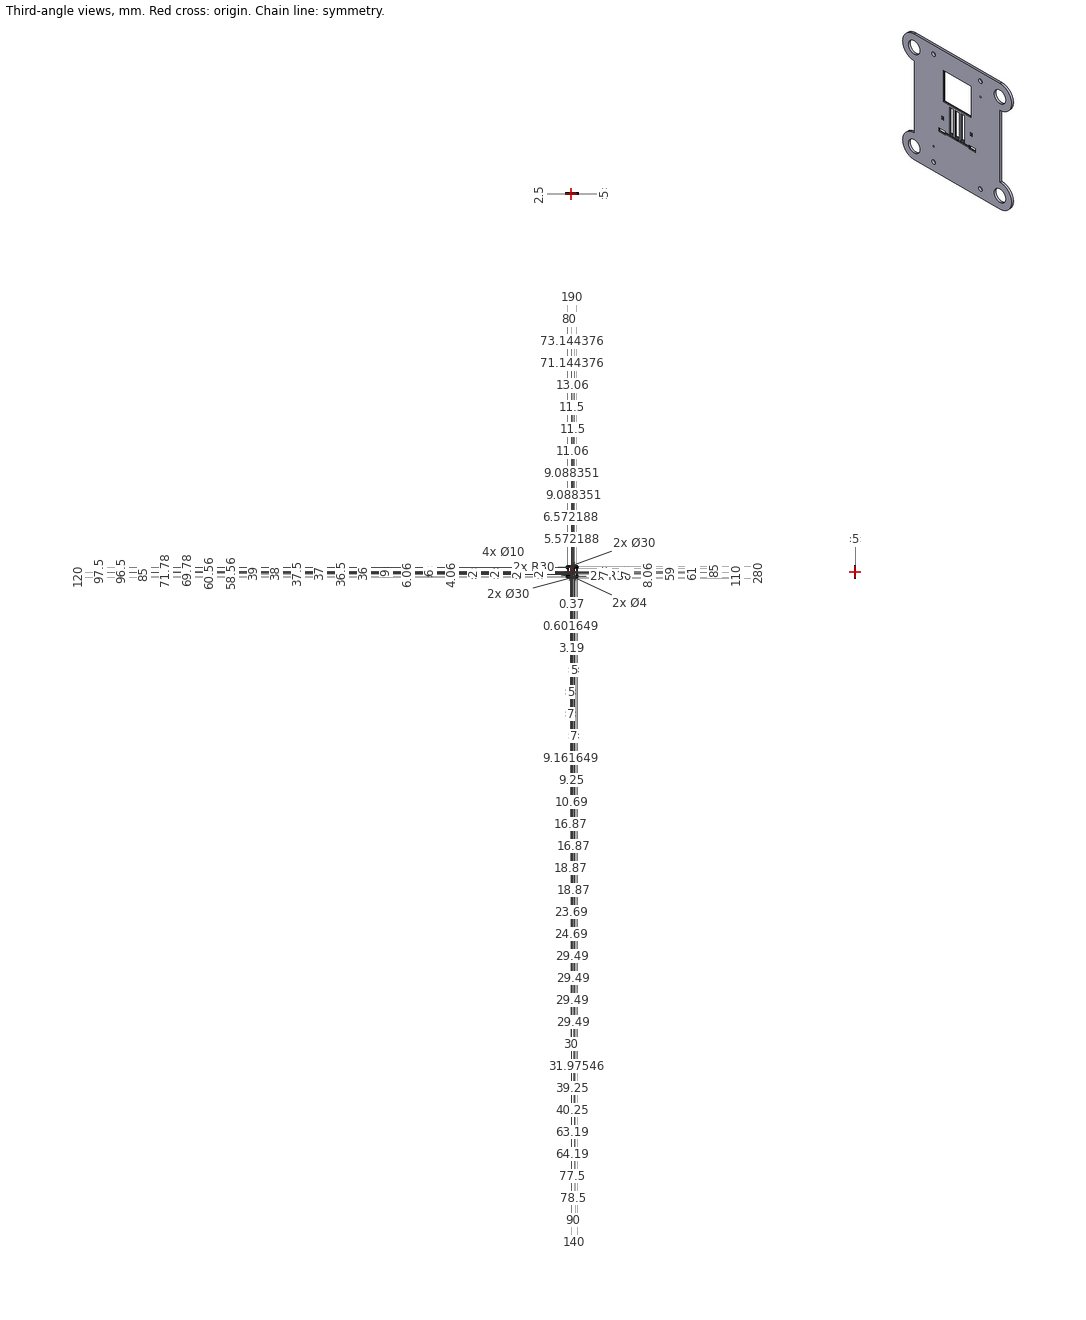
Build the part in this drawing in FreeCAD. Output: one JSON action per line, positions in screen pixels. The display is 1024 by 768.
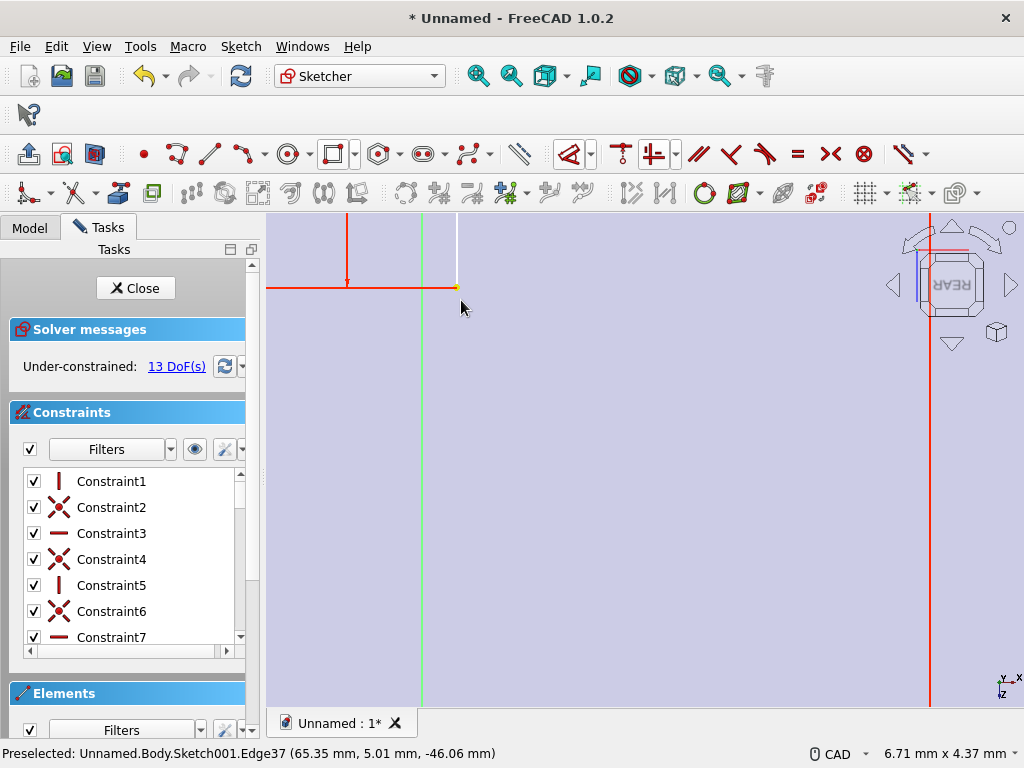
{"action": "left_click", "coordinate": [457, 288]}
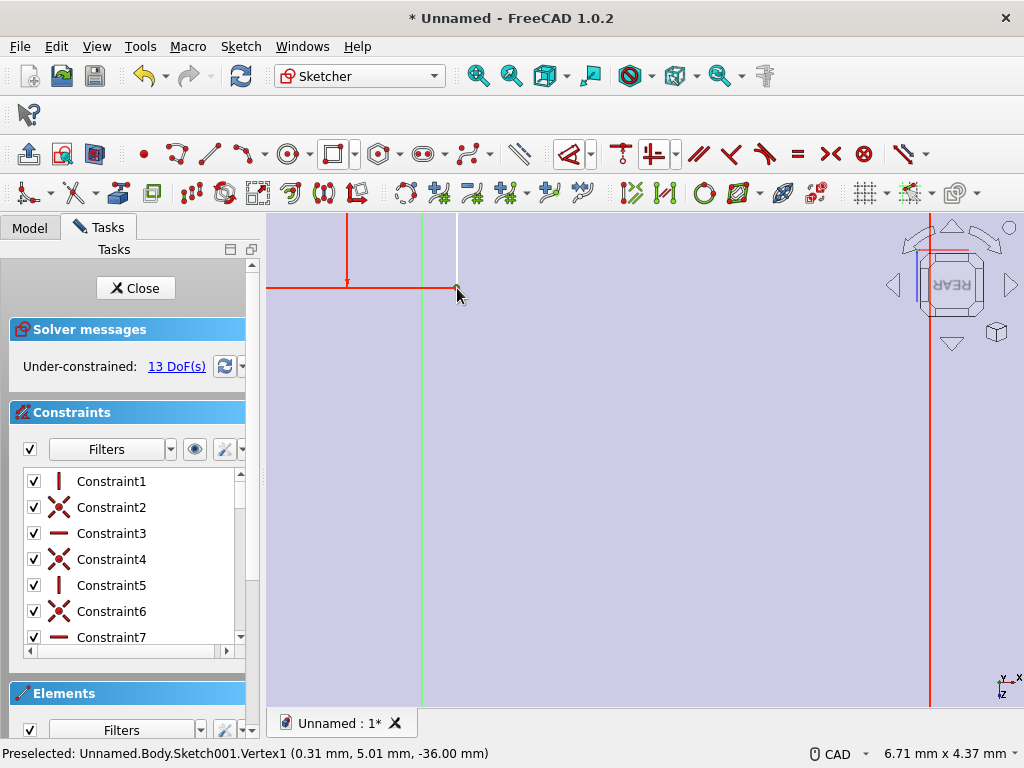
{"action": "left_click", "coordinate": [590, 154]}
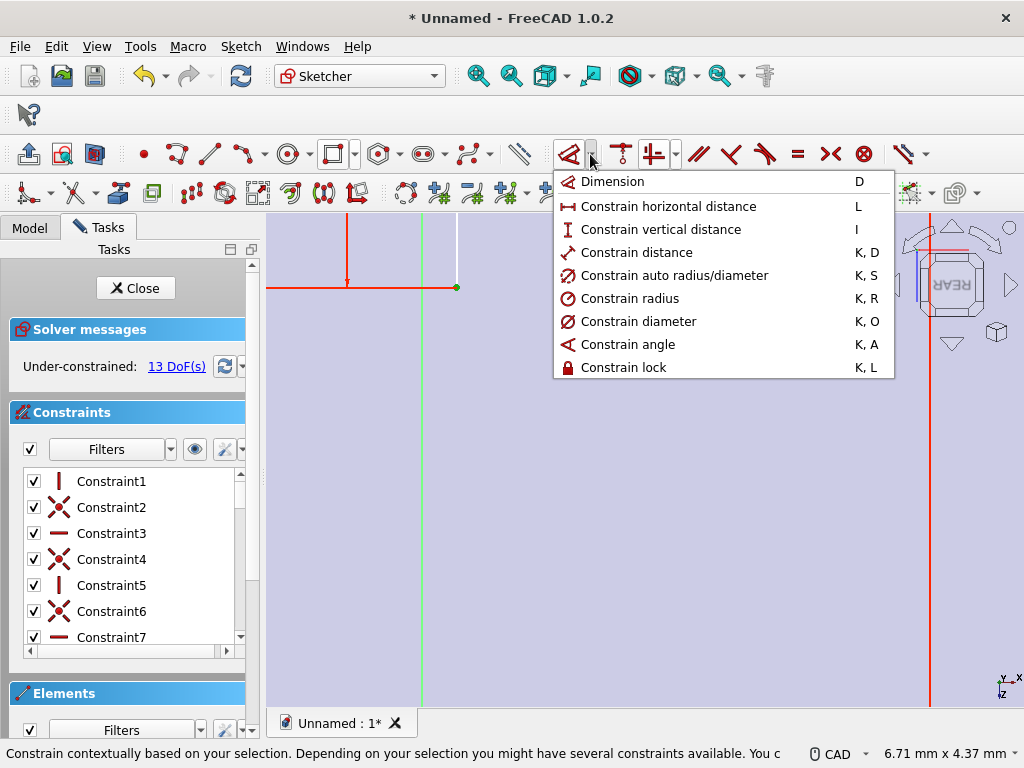
{"action": "left_click", "coordinate": [724, 206]}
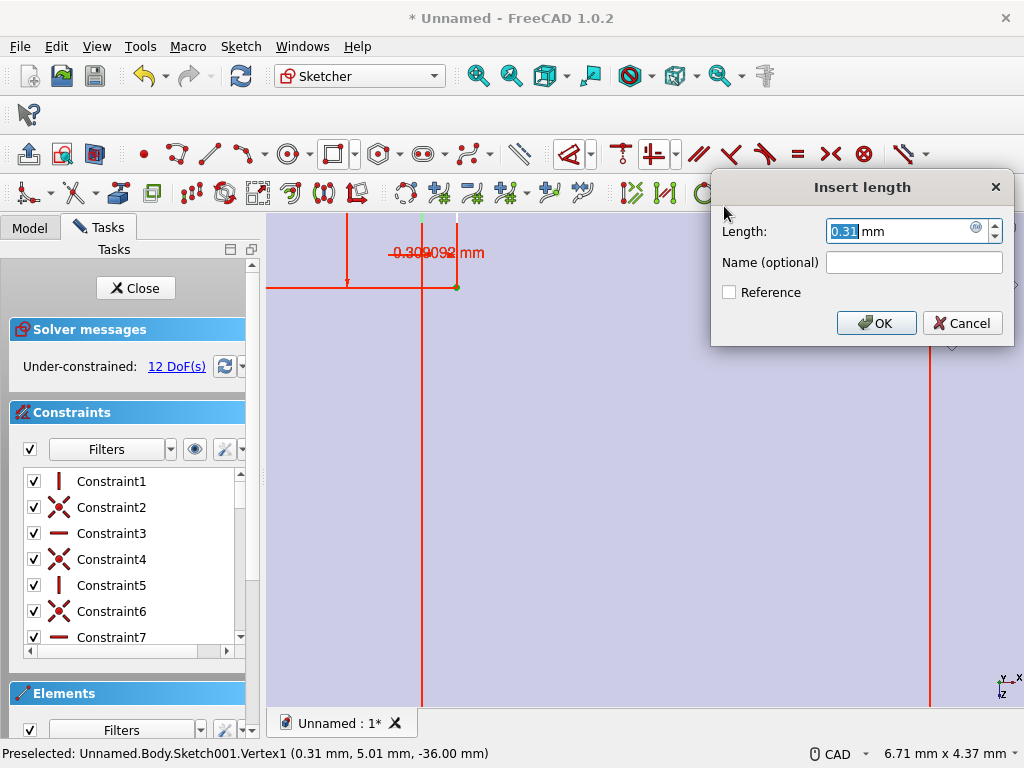
{"action": "type", "text": "0.37"}
{"action": "key", "text": "Return"}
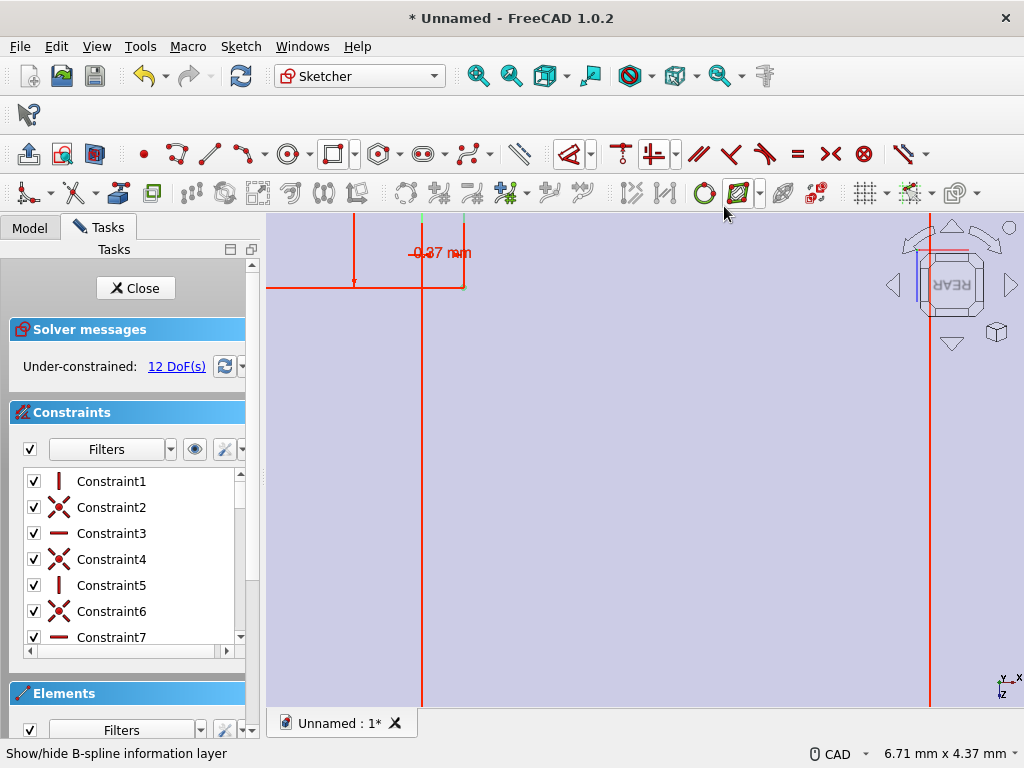
{"action": "scroll", "coordinate": [576, 460], "scroll_direction": "down", "scroll_amount": 15}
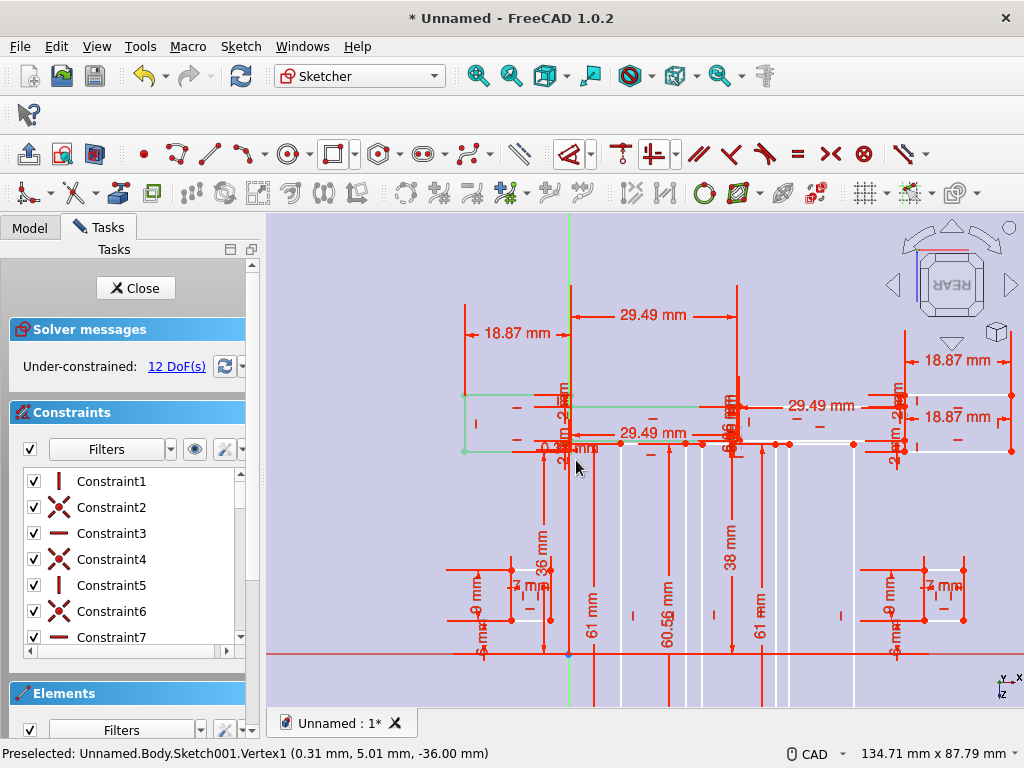
{"action": "scroll", "coordinate": [483, 263], "scroll_direction": "down", "scroll_amount": 5}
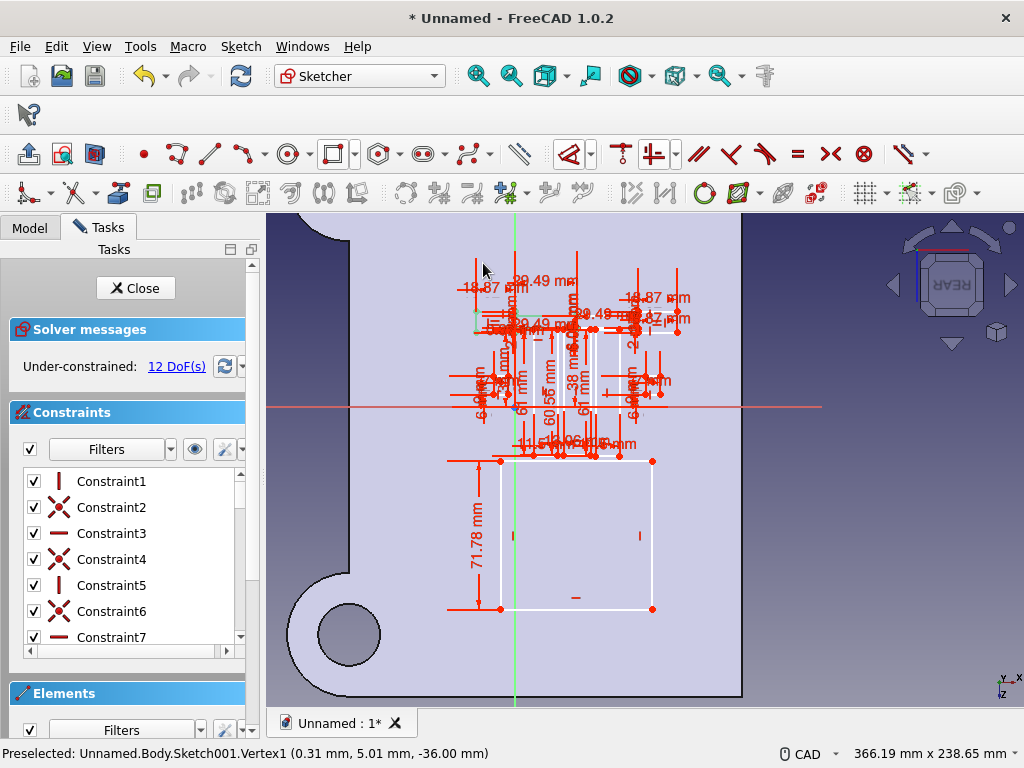
{"action": "left_click", "coordinate": [501, 610]}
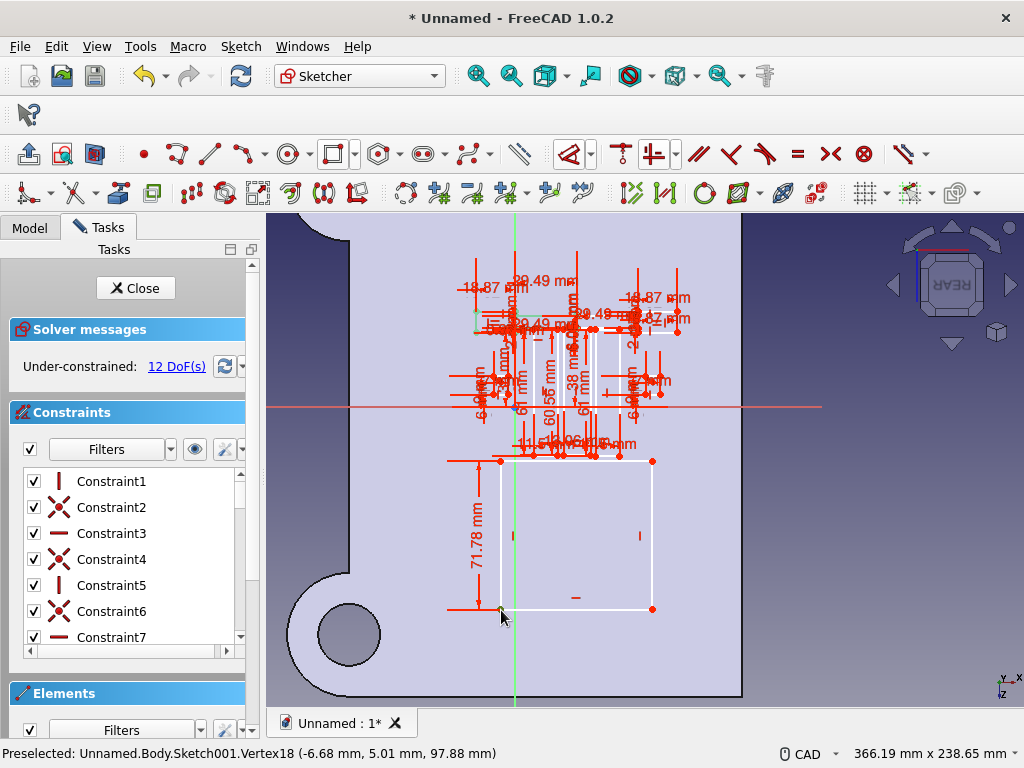
{"action": "left_click", "coordinate": [590, 154]}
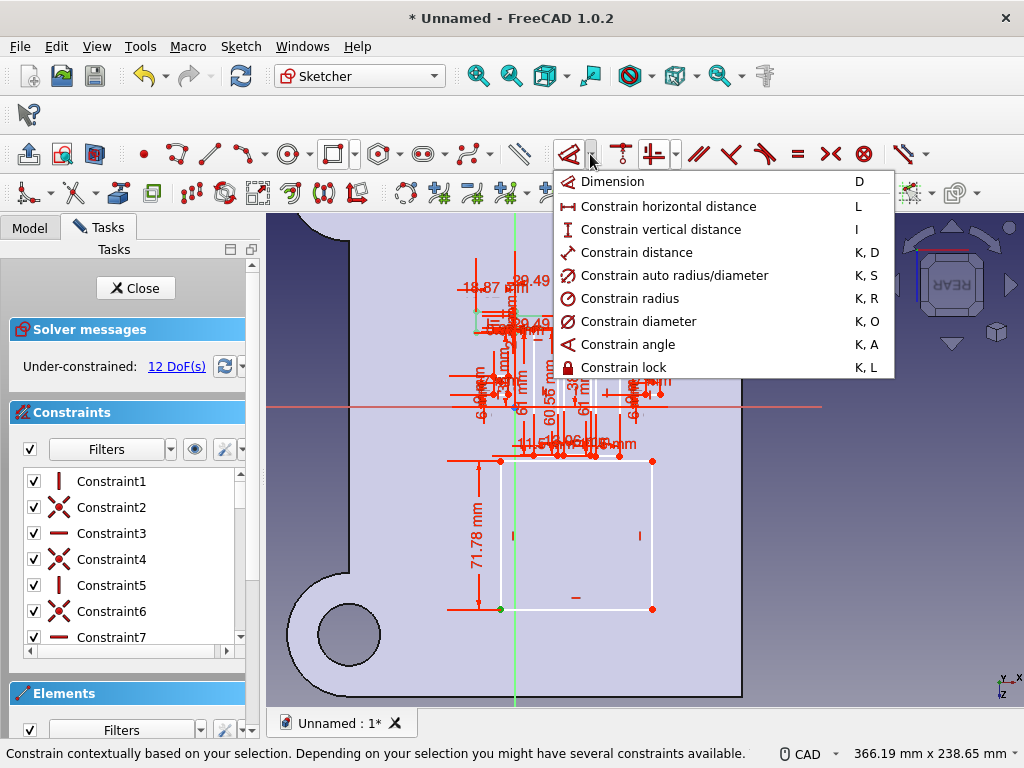
{"action": "left_click", "coordinate": [724, 230]}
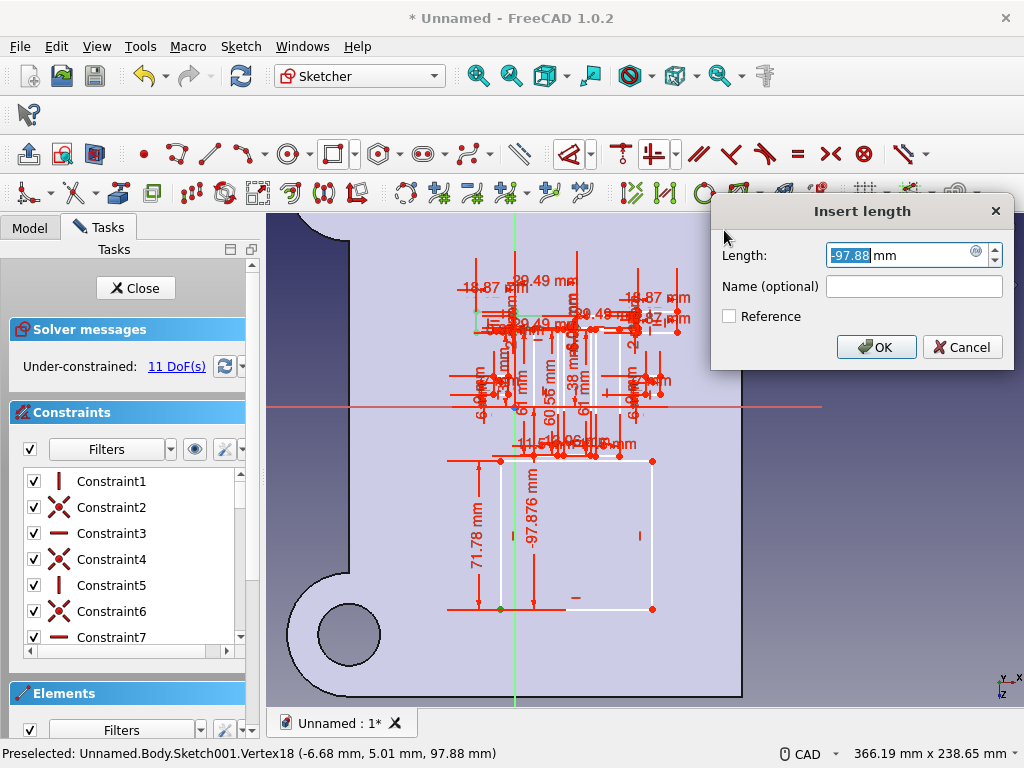
{"action": "type", "text": "-97.5"}
{"action": "key", "text": "Return"}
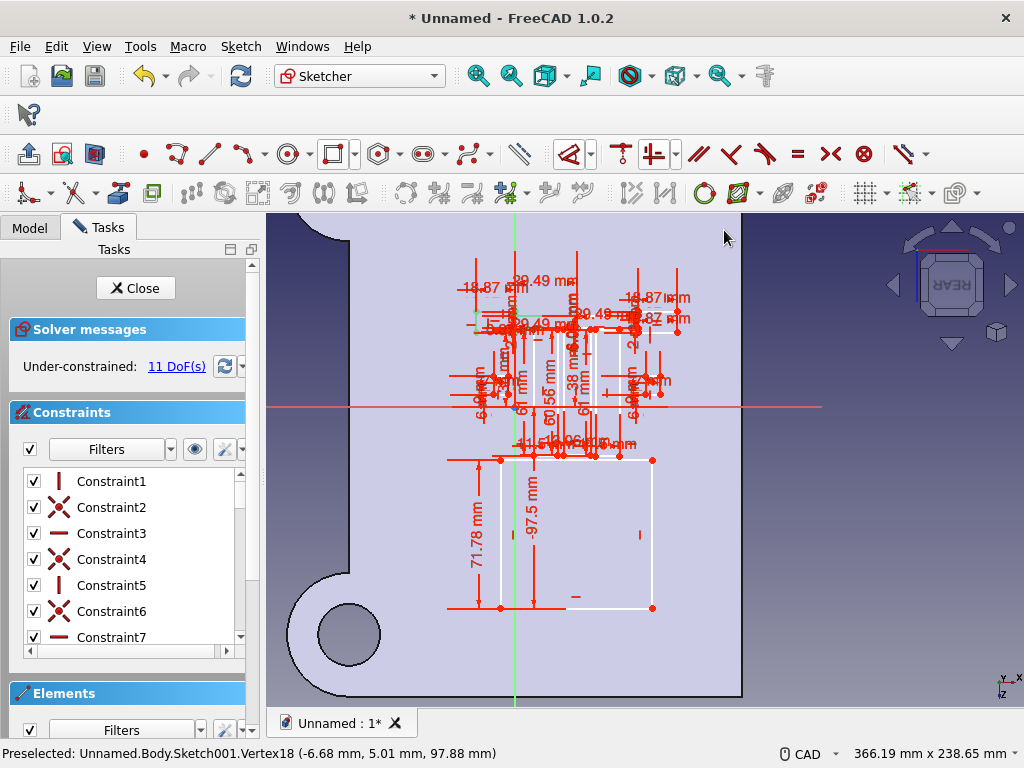
{"action": "scroll", "coordinate": [508, 395], "scroll_direction": "up", "scroll_amount": 9}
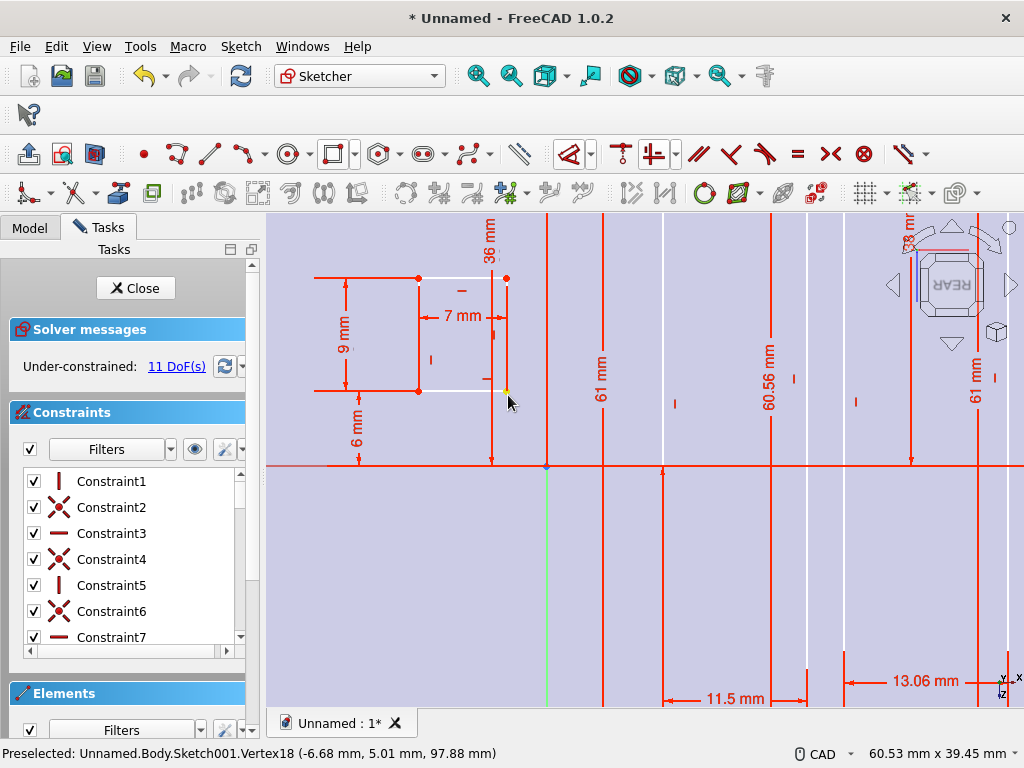
{"action": "left_click", "coordinate": [507, 391]}